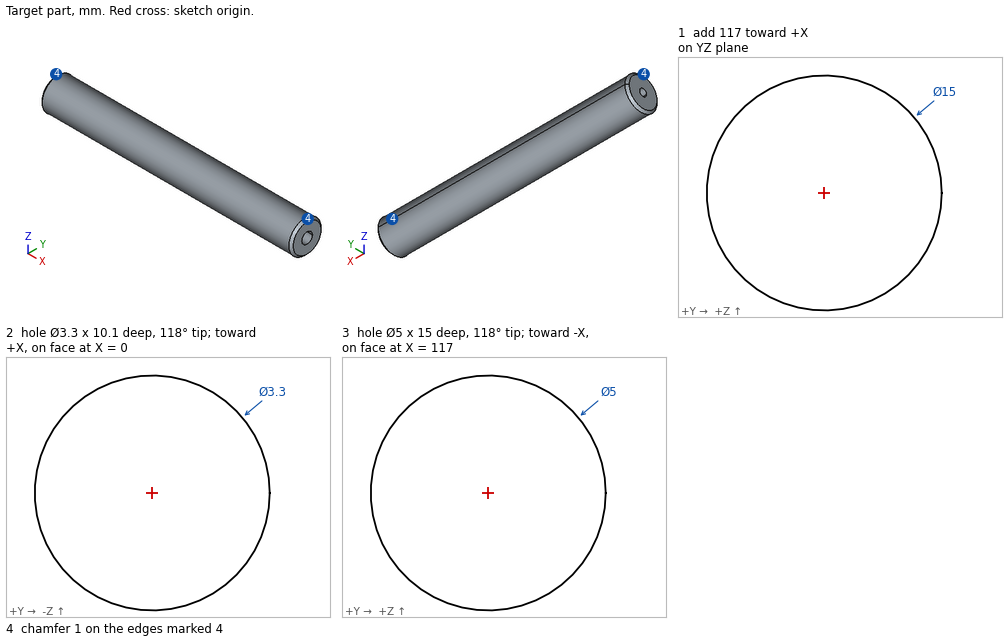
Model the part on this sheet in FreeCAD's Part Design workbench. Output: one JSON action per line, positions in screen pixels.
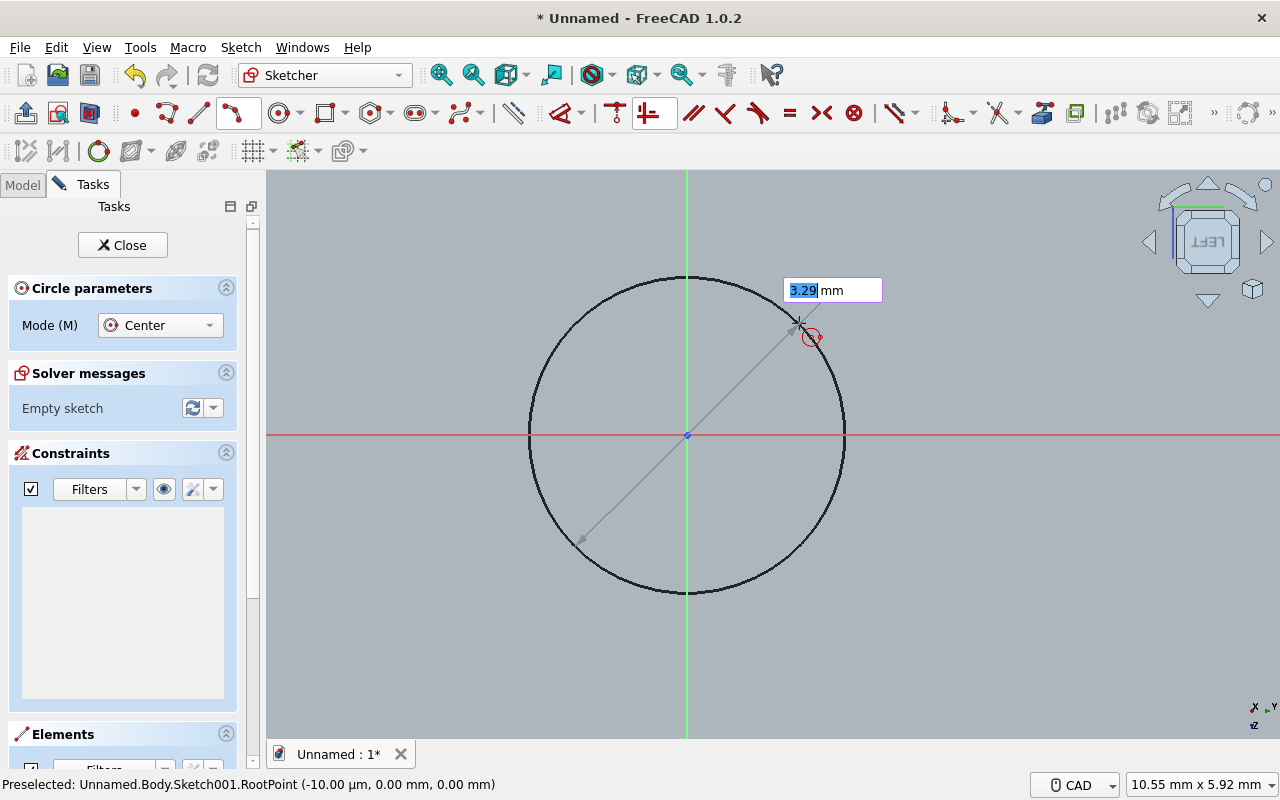
{"action": "type", "text": "3.3"}
{"action": "key", "text": "Return"}
{"action": "key", "text": "Escape"}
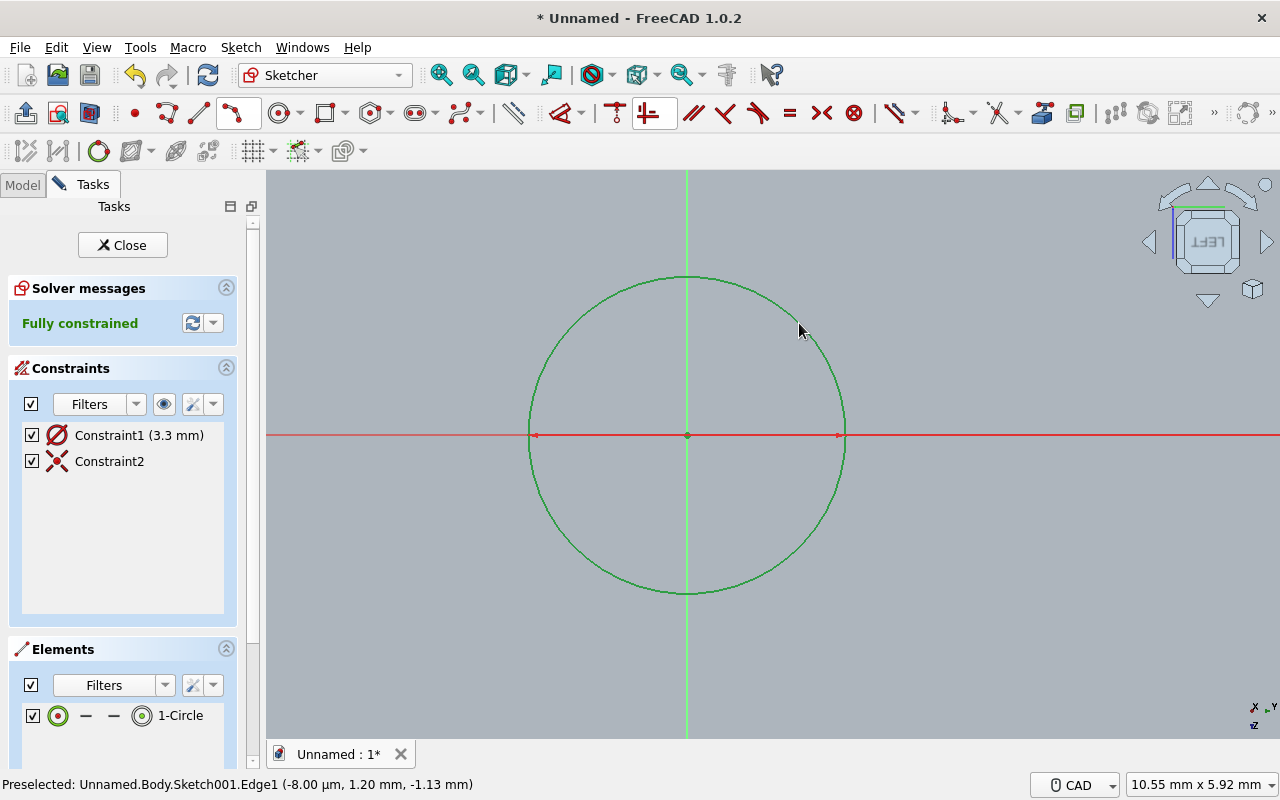
{"action": "left_click", "coordinate": [123, 245]}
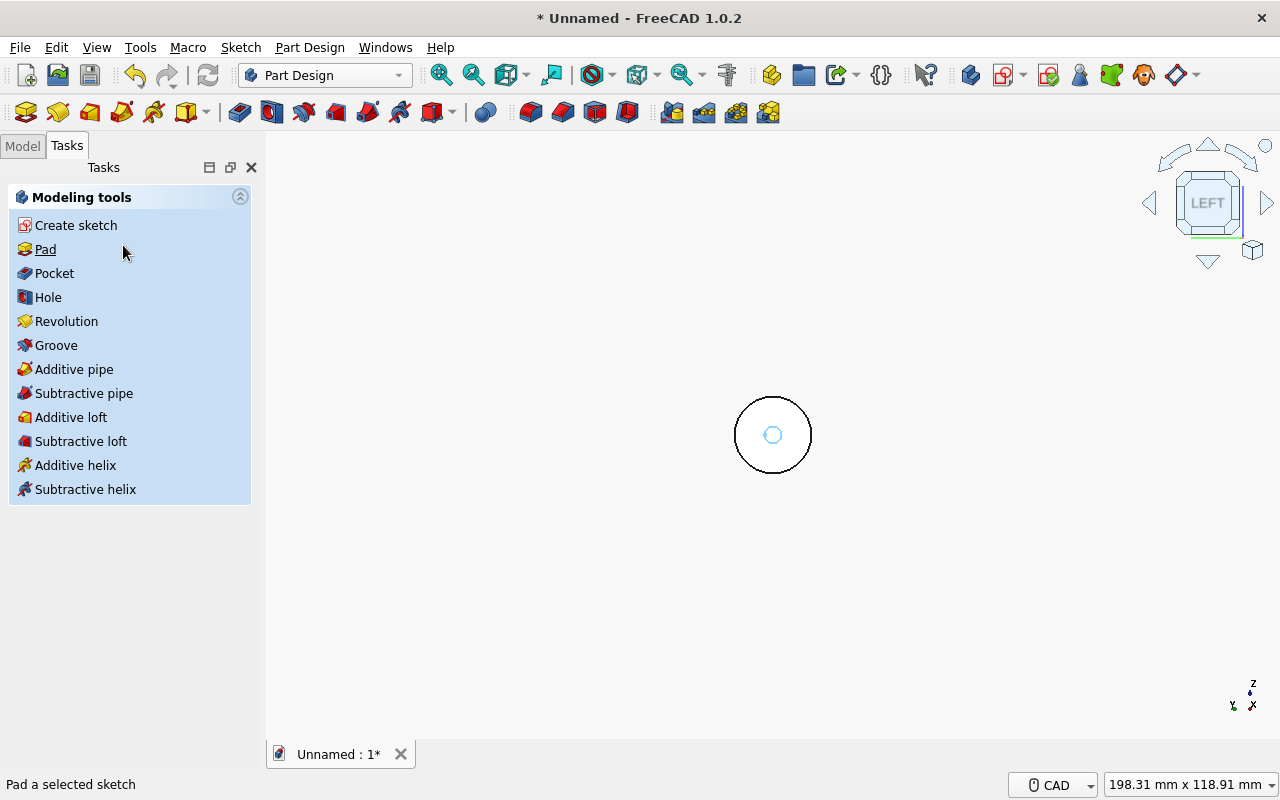
{"action": "left_click", "coordinate": [272, 112]}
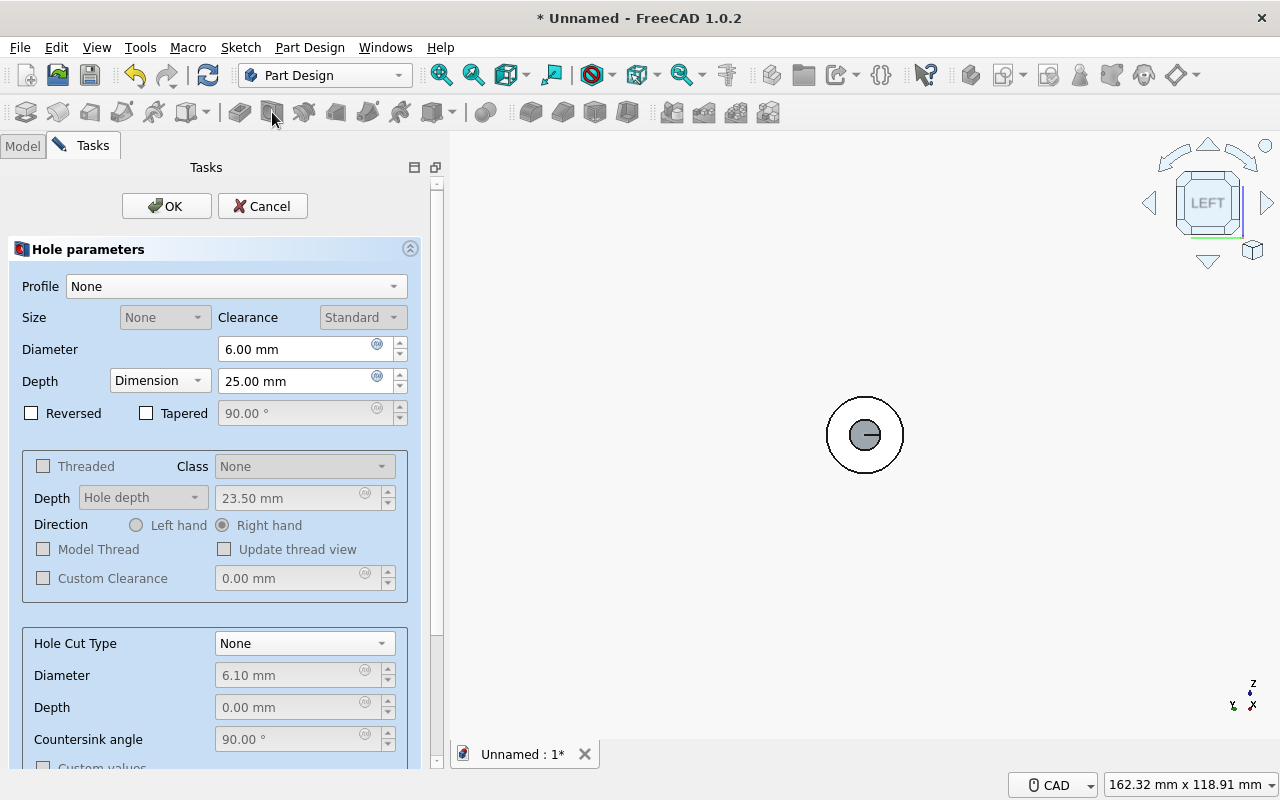
{"action": "triple_click", "coordinate": [305, 349]}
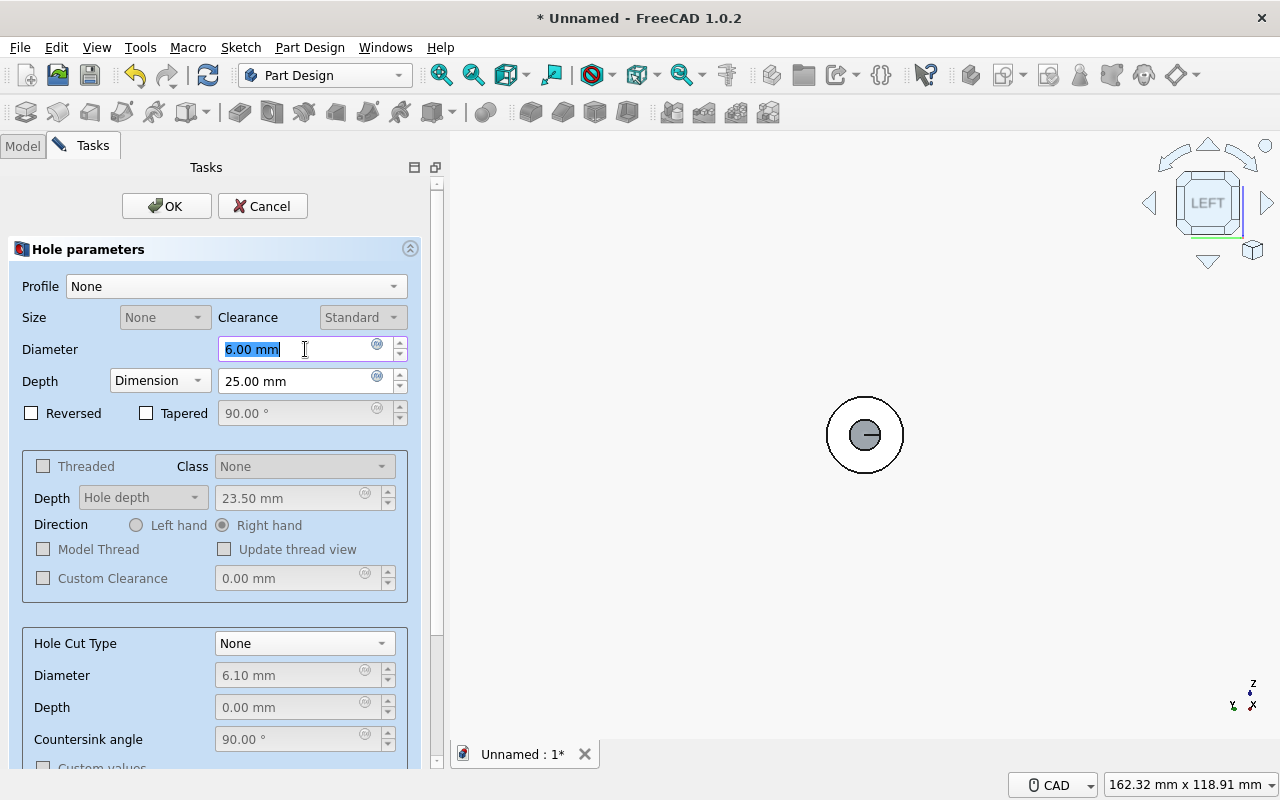
{"action": "type", "text": "3.3"}
{"action": "key", "text": "Tab"}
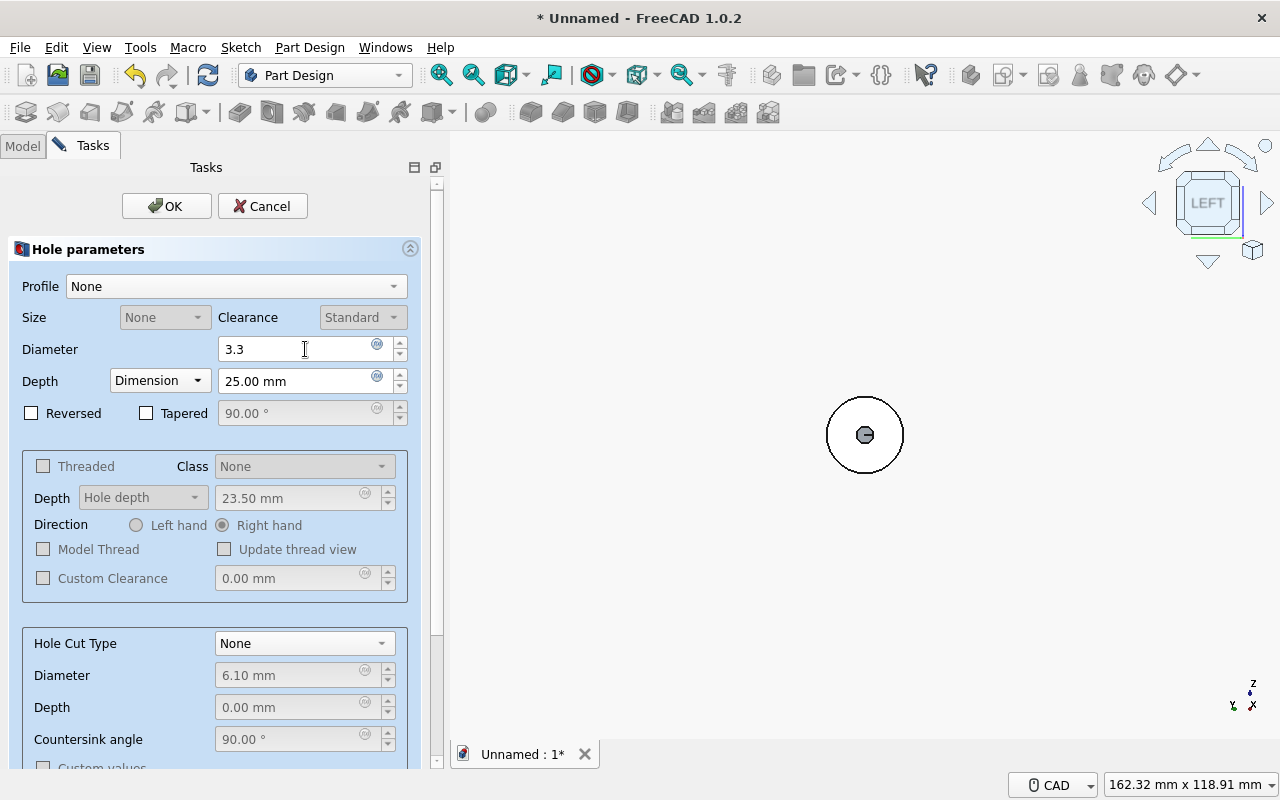
{"action": "triple_click", "coordinate": [305, 381]}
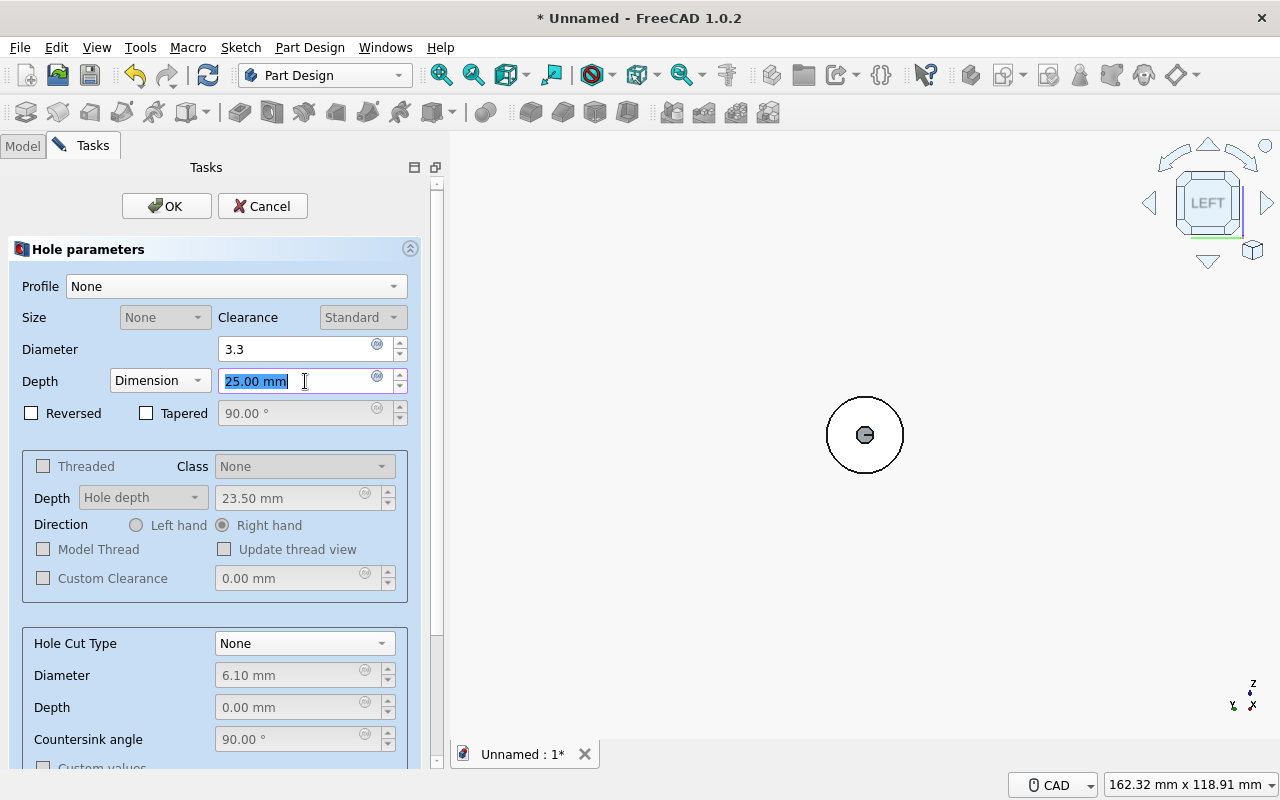
{"action": "type", "text": "10.1"}
{"action": "key", "text": "Tab"}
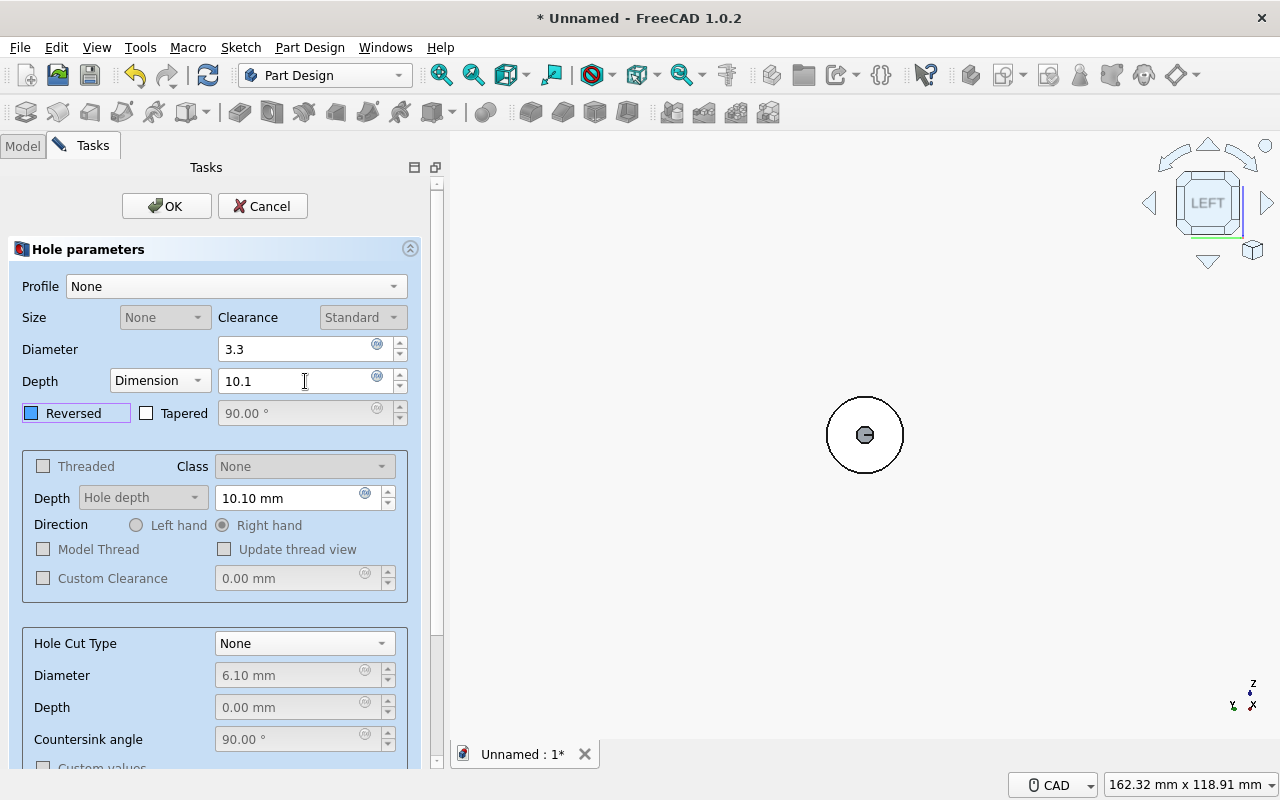
{"action": "left_click", "coordinate": [167, 206]}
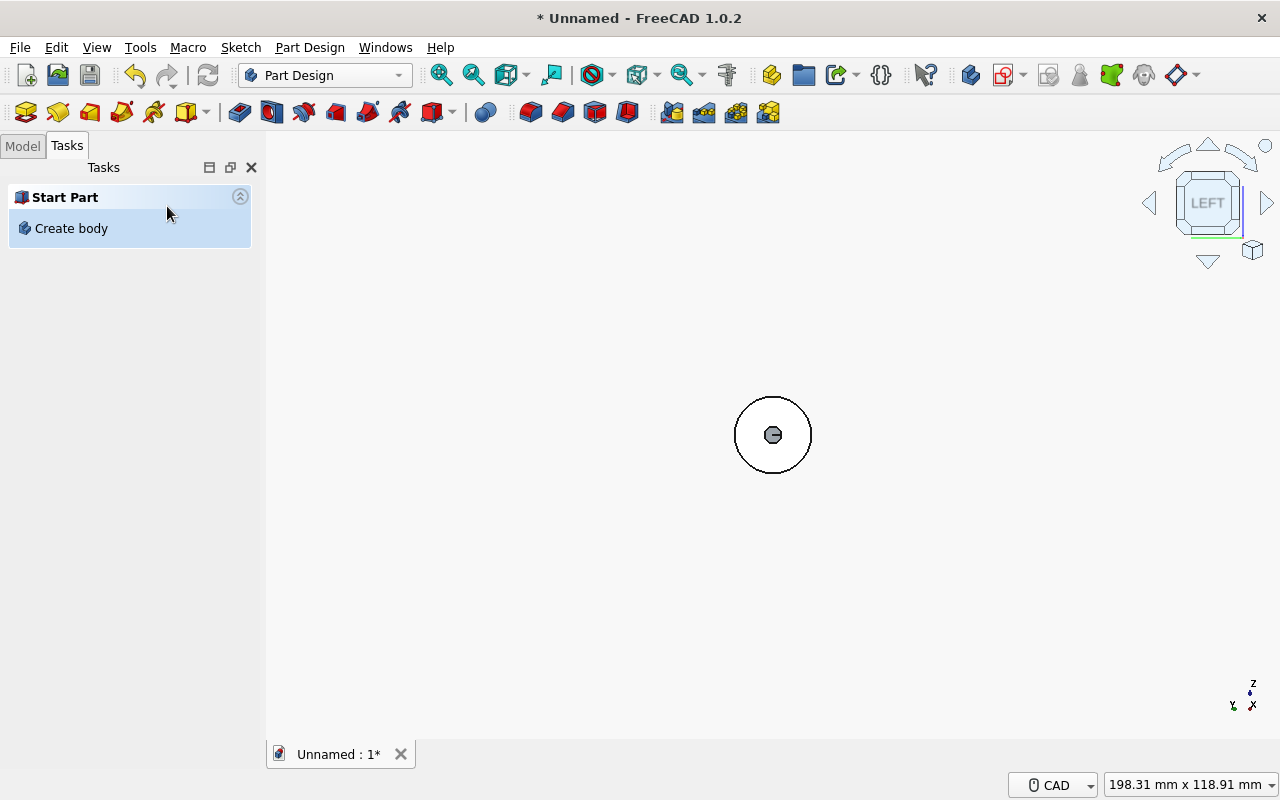
{"action": "left_click", "coordinate": [442, 76]}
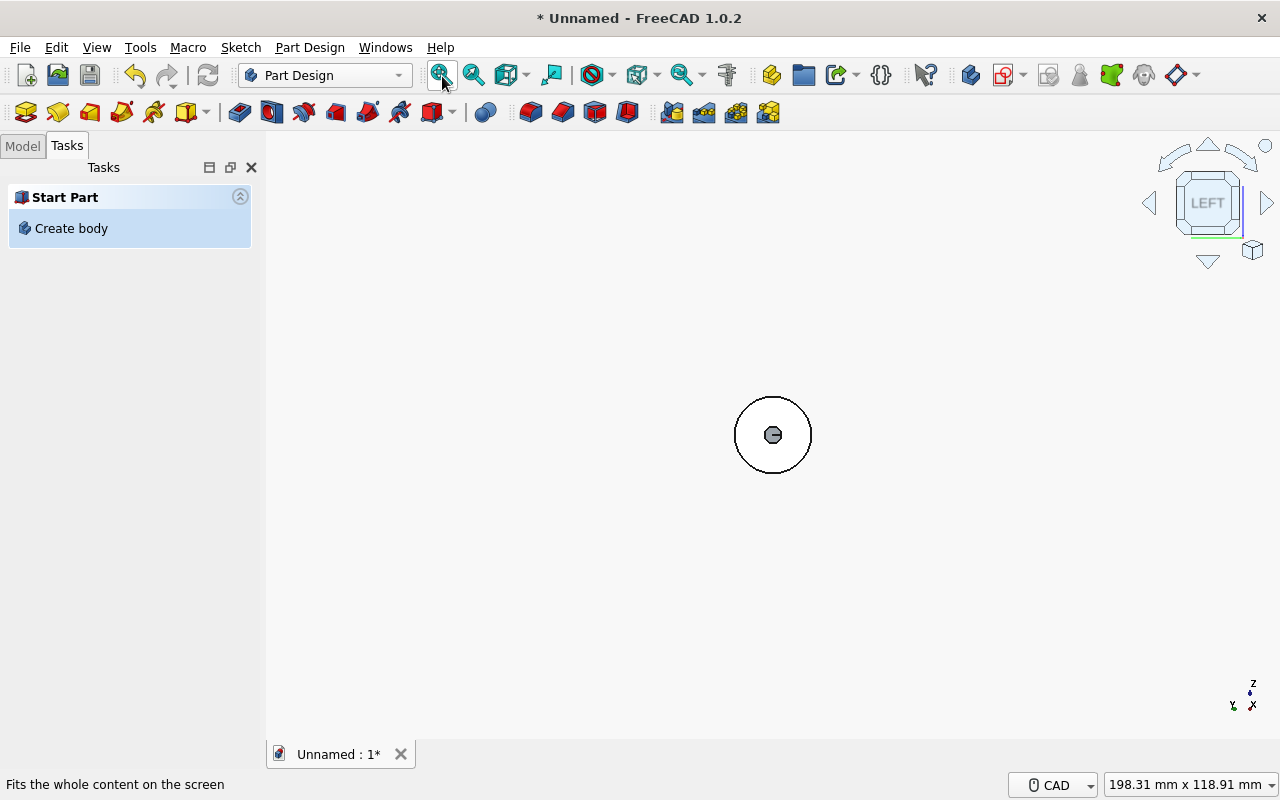
{"action": "key", "text": "0"}